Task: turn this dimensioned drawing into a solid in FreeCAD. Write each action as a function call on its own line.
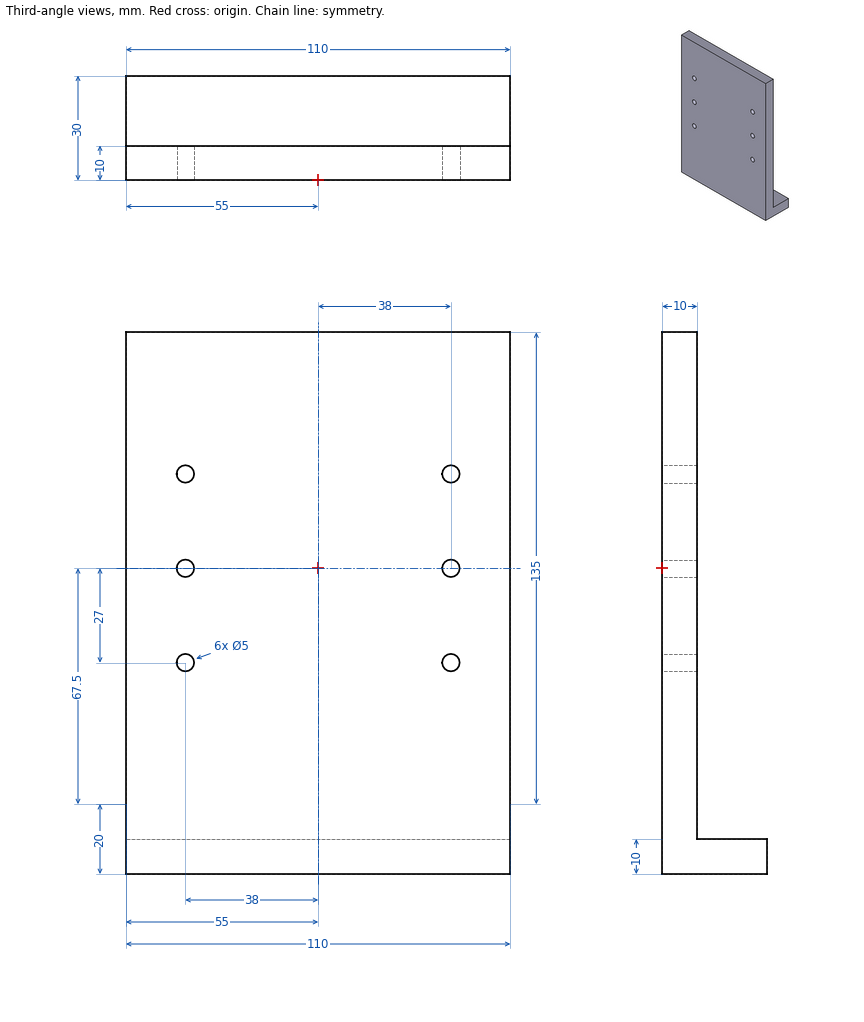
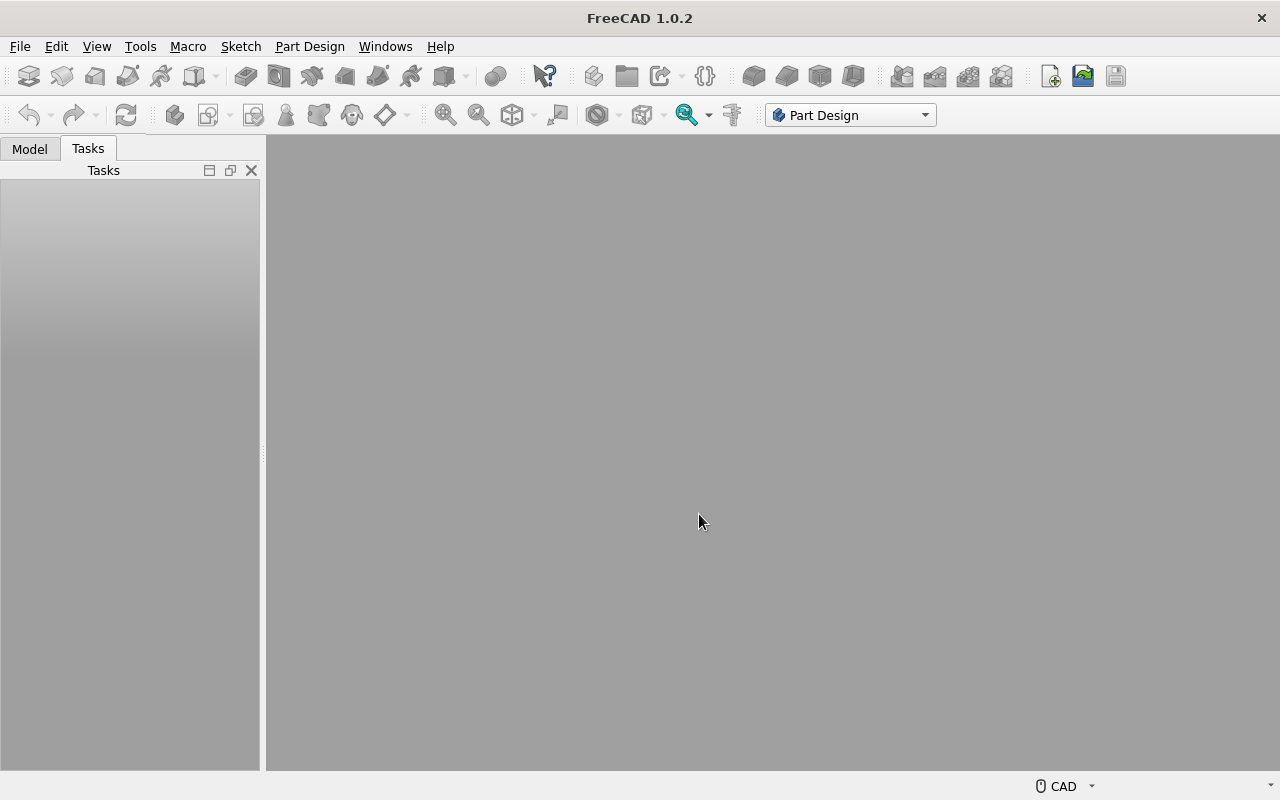
click(1050, 76)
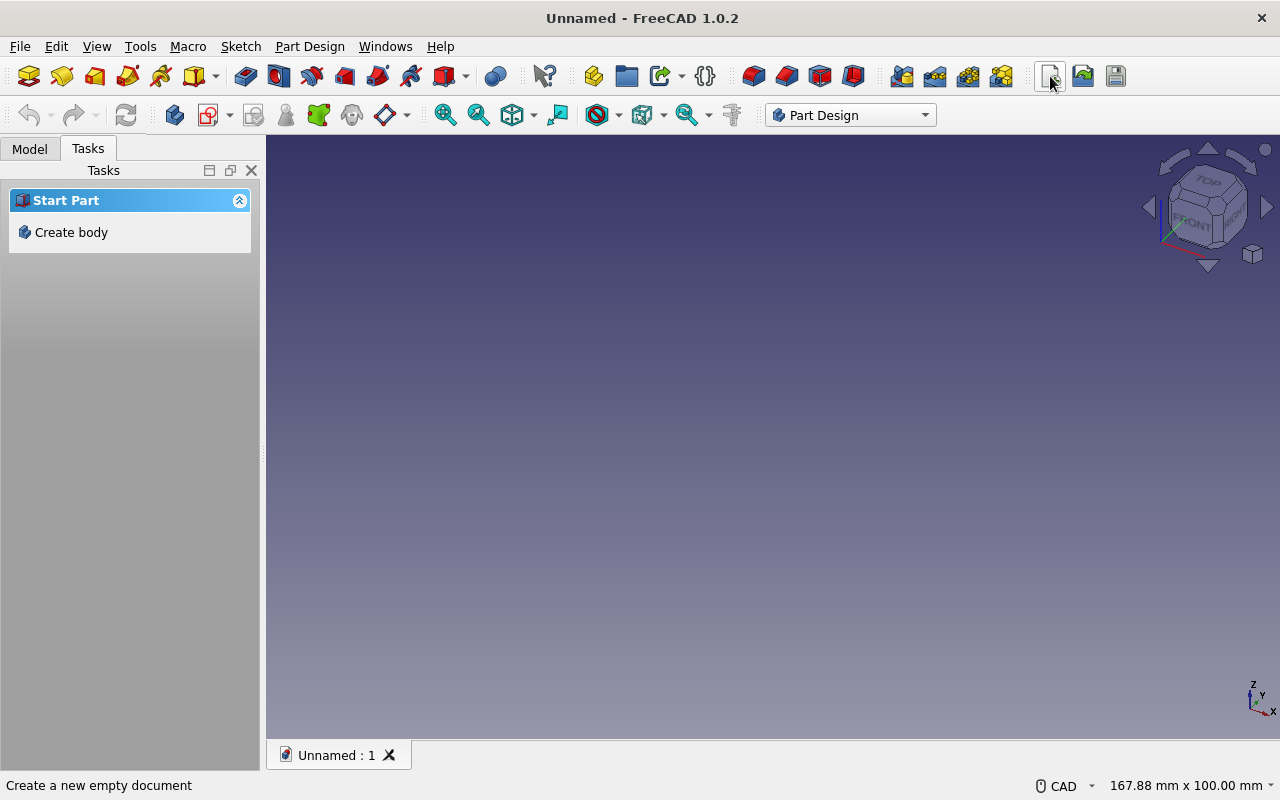
click(208, 116)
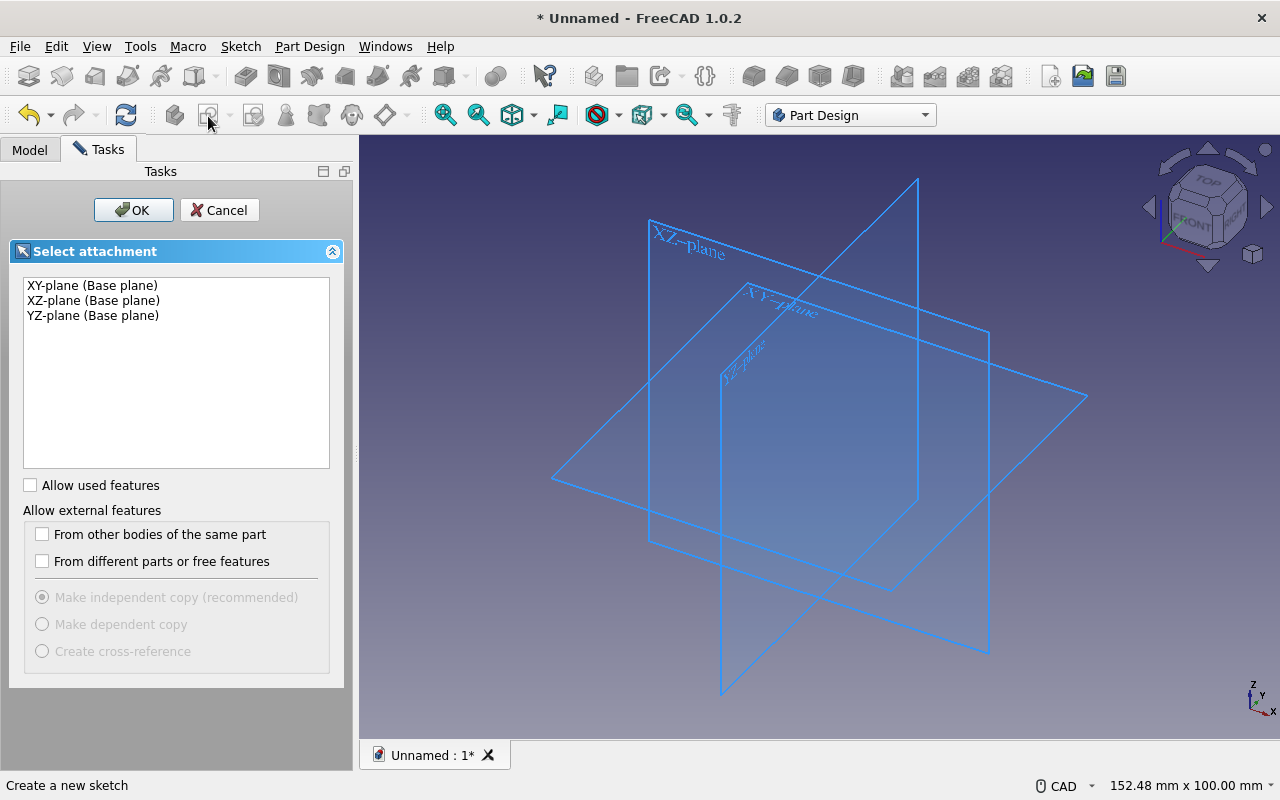
click(84, 300)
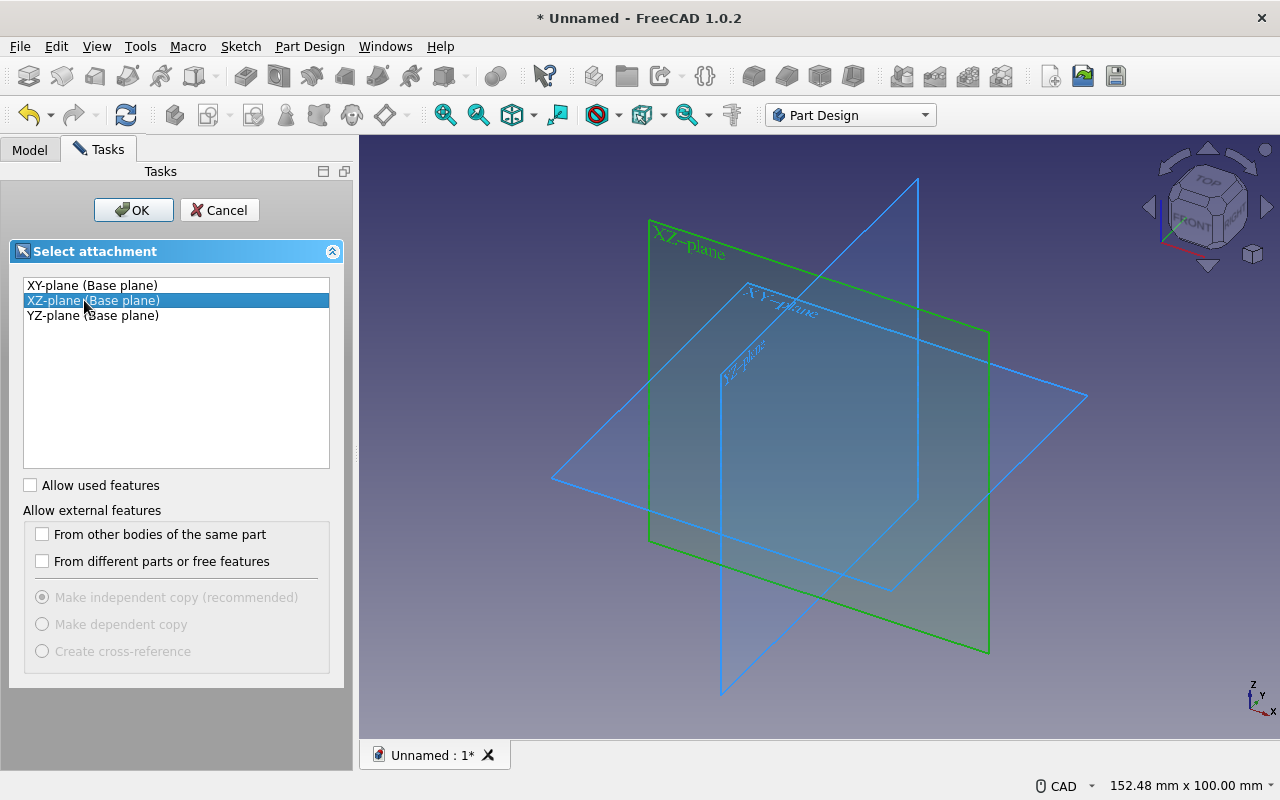
click(134, 210)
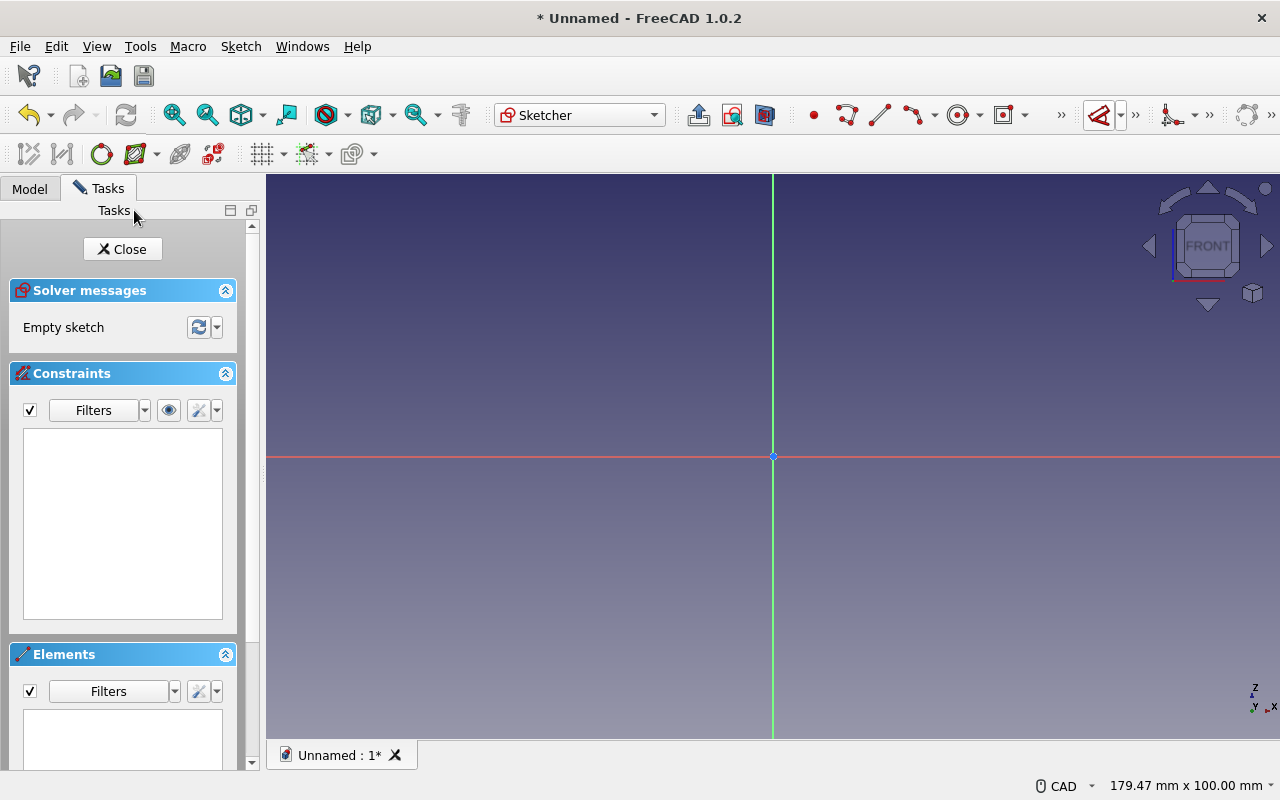
scroll(649, 456, down, 4)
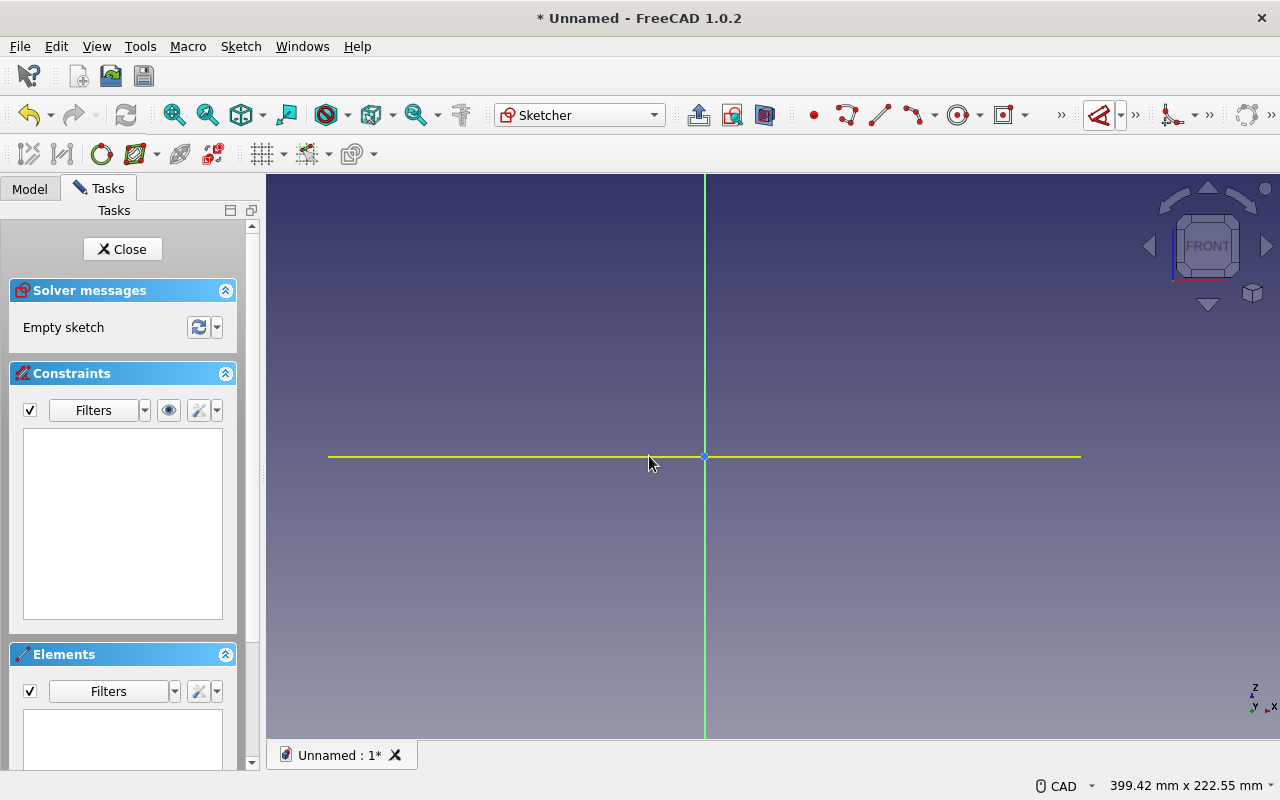
click(1002, 116)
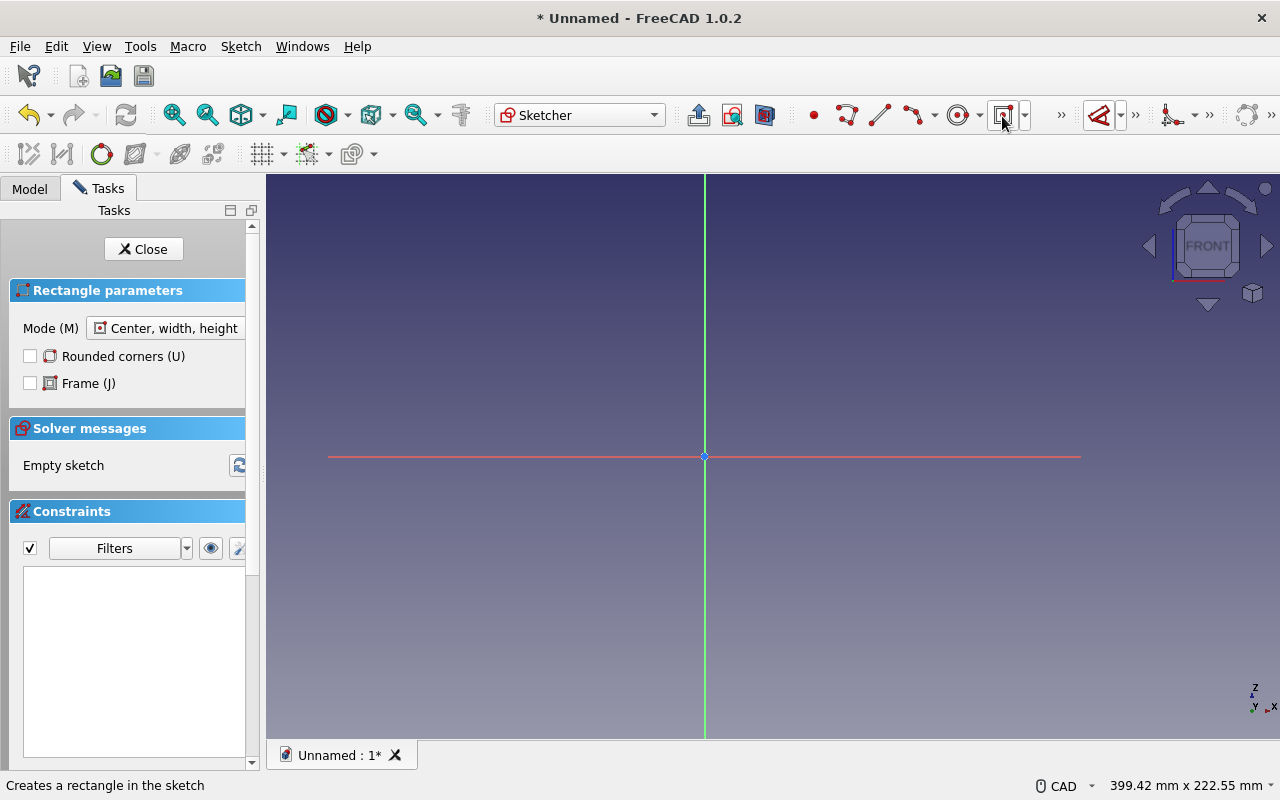
click(705, 456)
click(845, 285)
key(Escape)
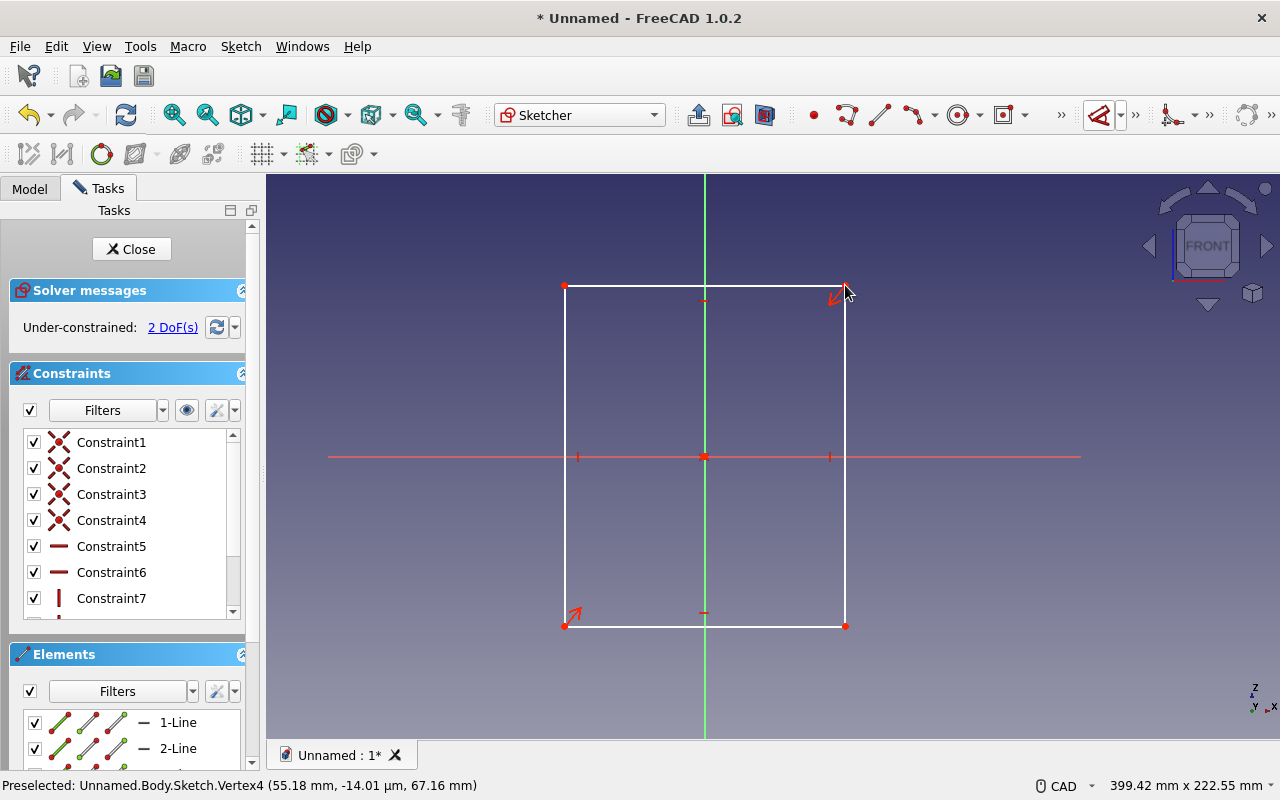
click(1098, 116)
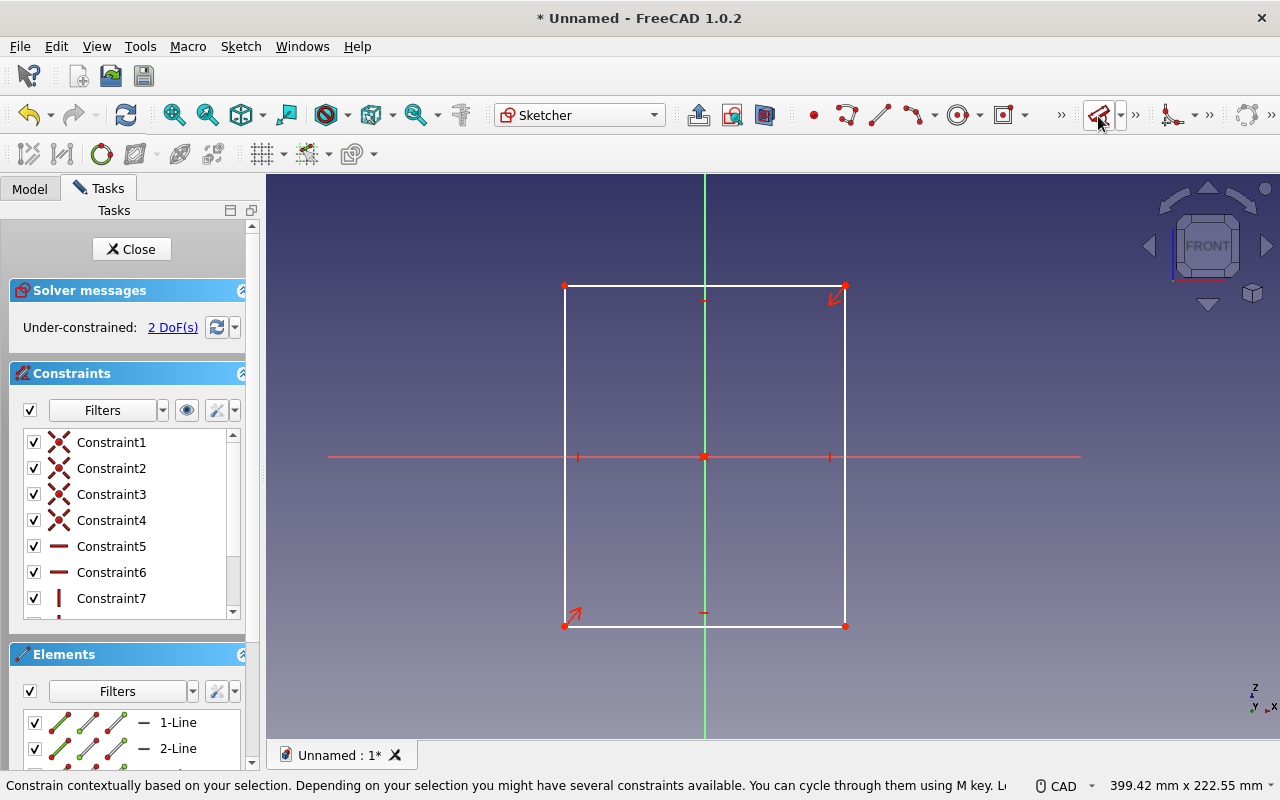
click(649, 627)
click(640, 661)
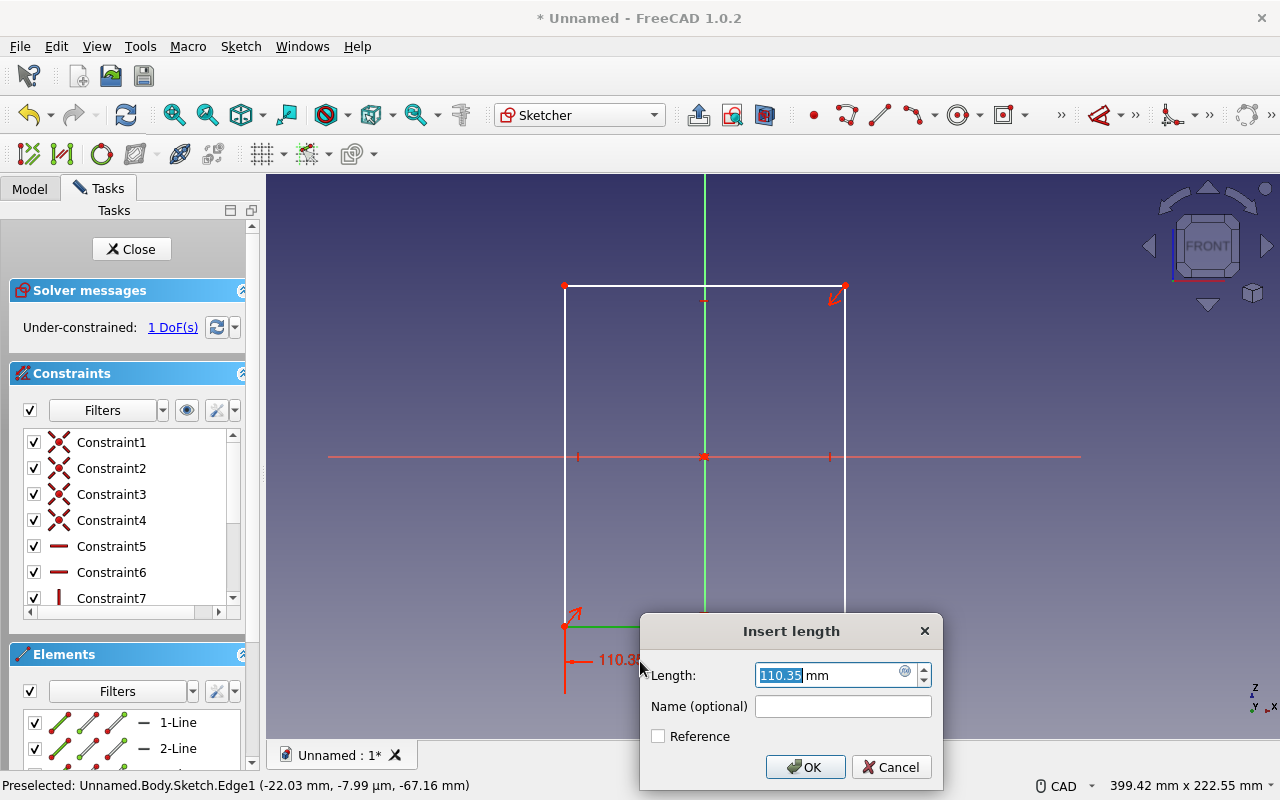
text(110)
key(Return)